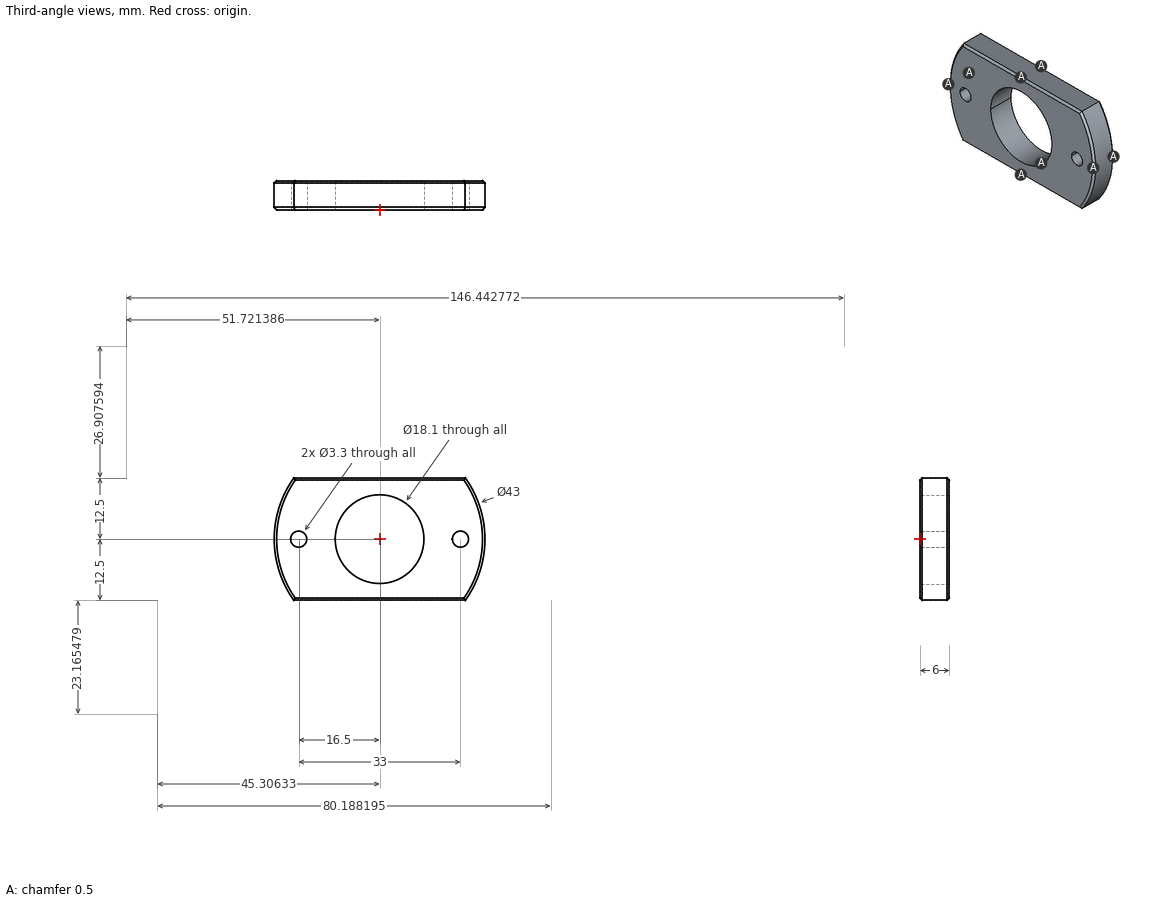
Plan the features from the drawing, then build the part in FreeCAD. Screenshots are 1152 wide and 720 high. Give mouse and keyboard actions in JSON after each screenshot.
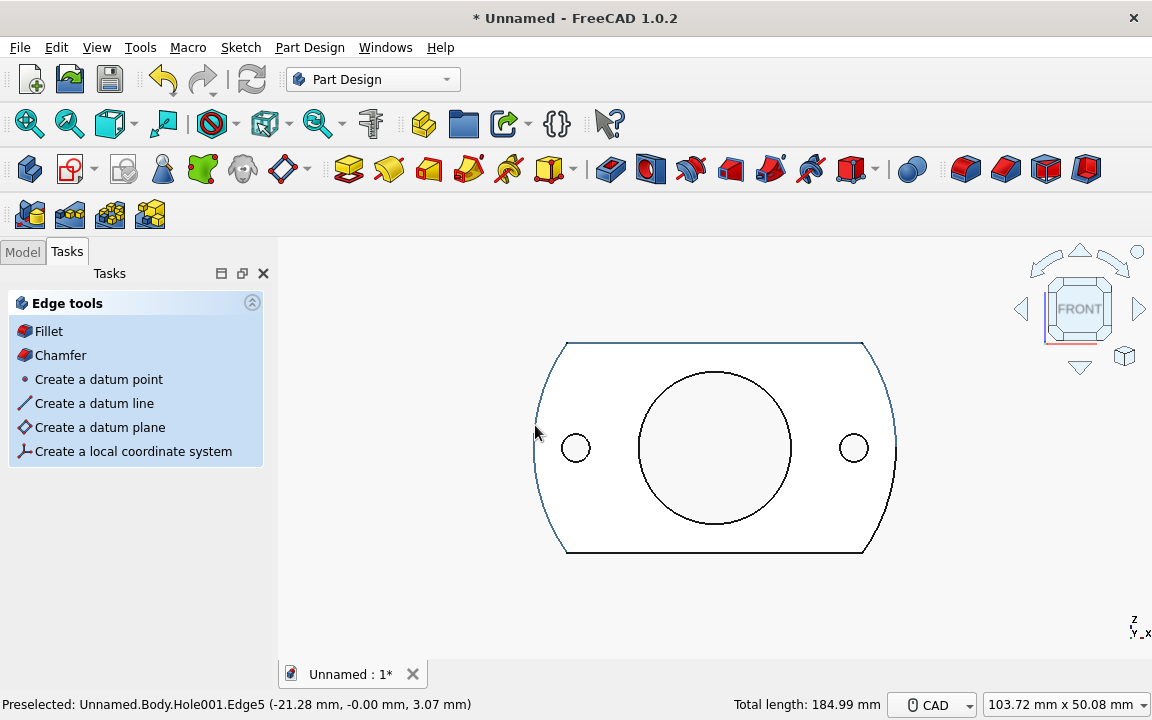
{"action": "key", "text": "3"}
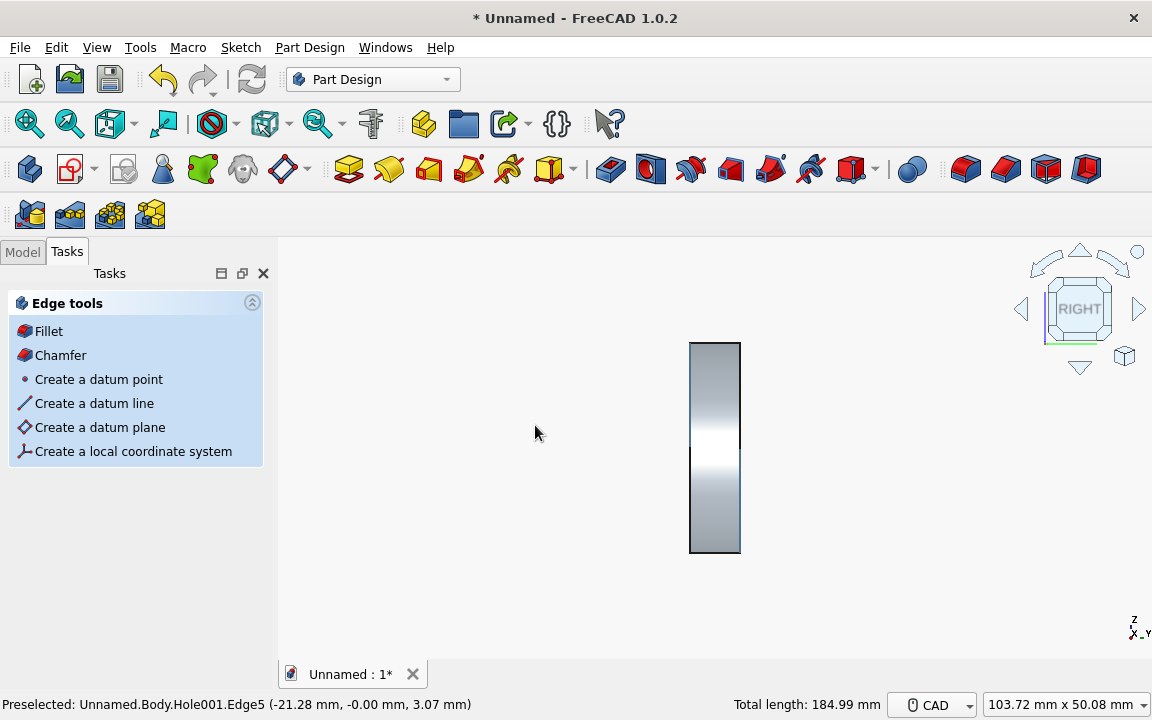
{"action": "key", "text": "5"}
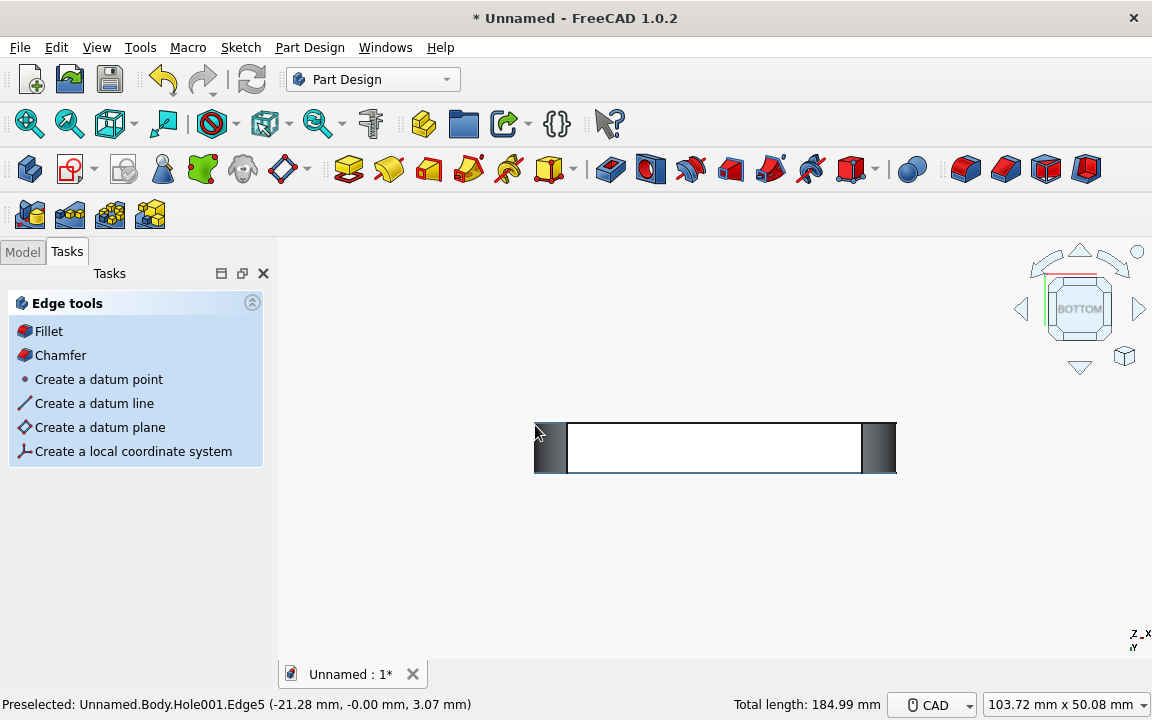
{"action": "left_click", "coordinate": [30, 124]}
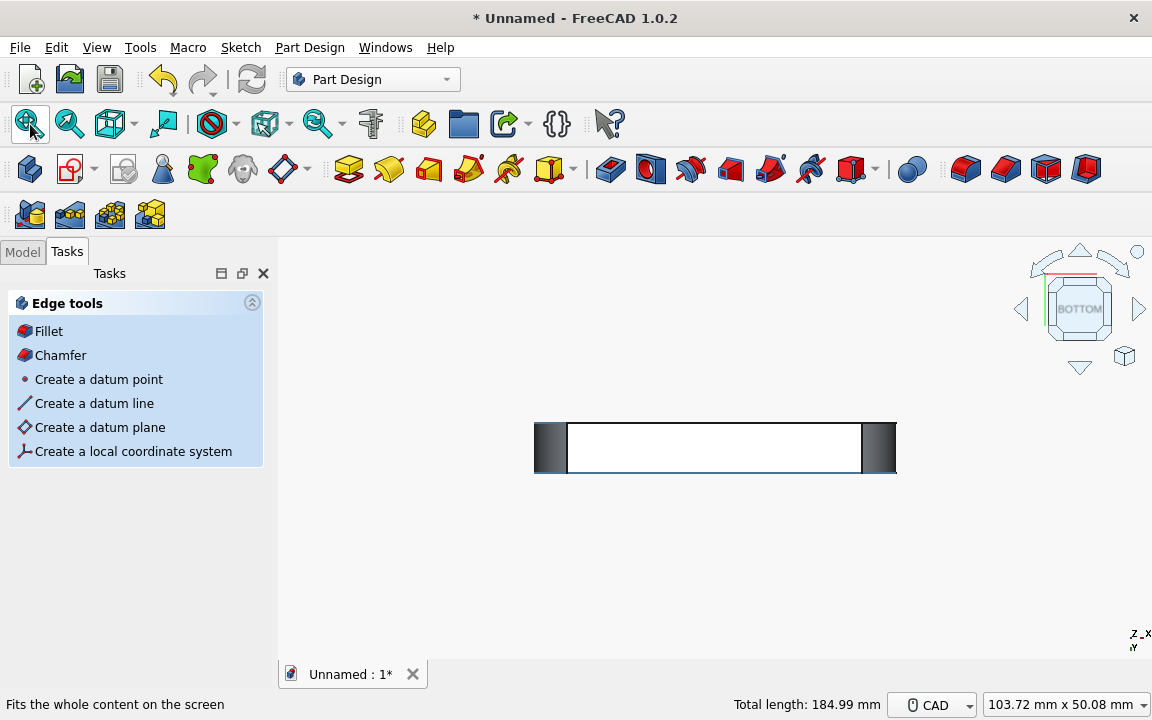
{"action": "left_click", "coordinate": [715, 422], "text": "ctrl"}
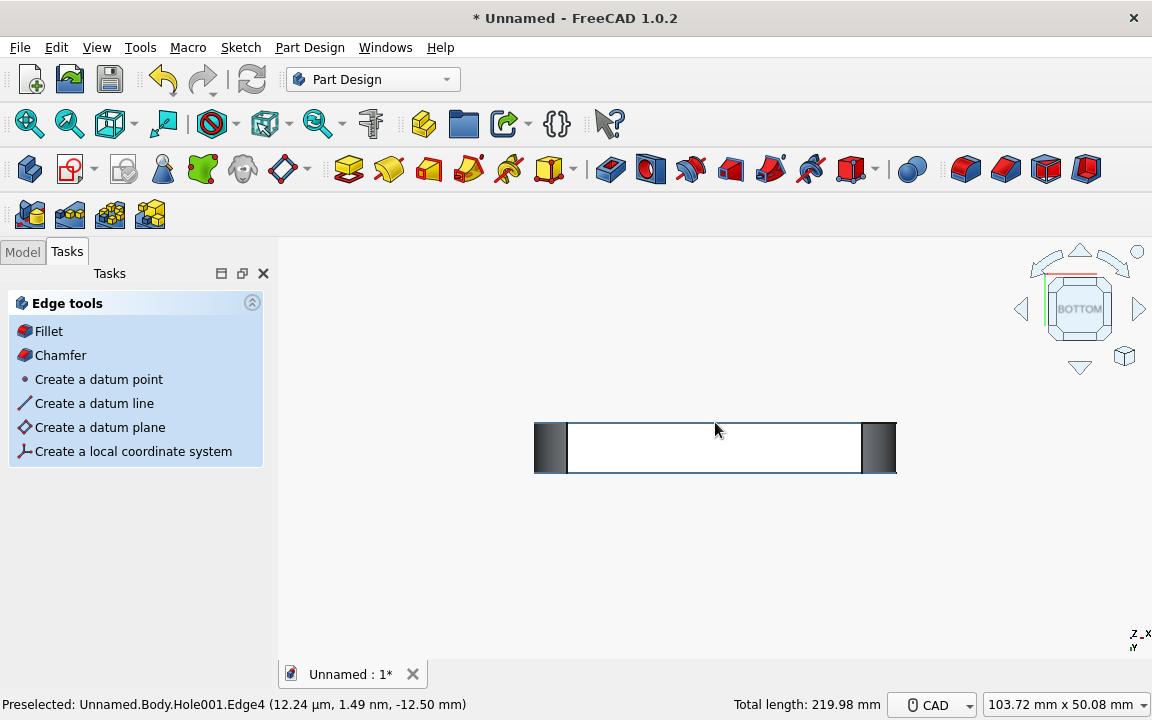
{"action": "left_click", "coordinate": [1006, 170]}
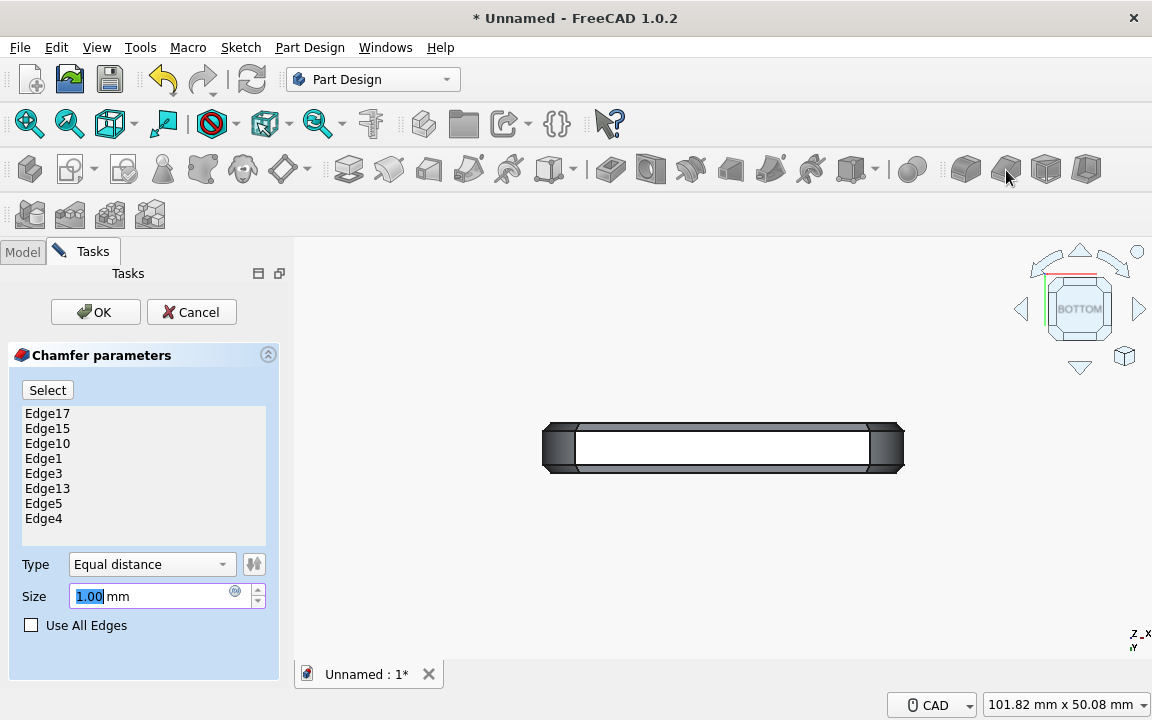
{"action": "type", "text": "0.5"}
{"action": "key", "text": "Tab"}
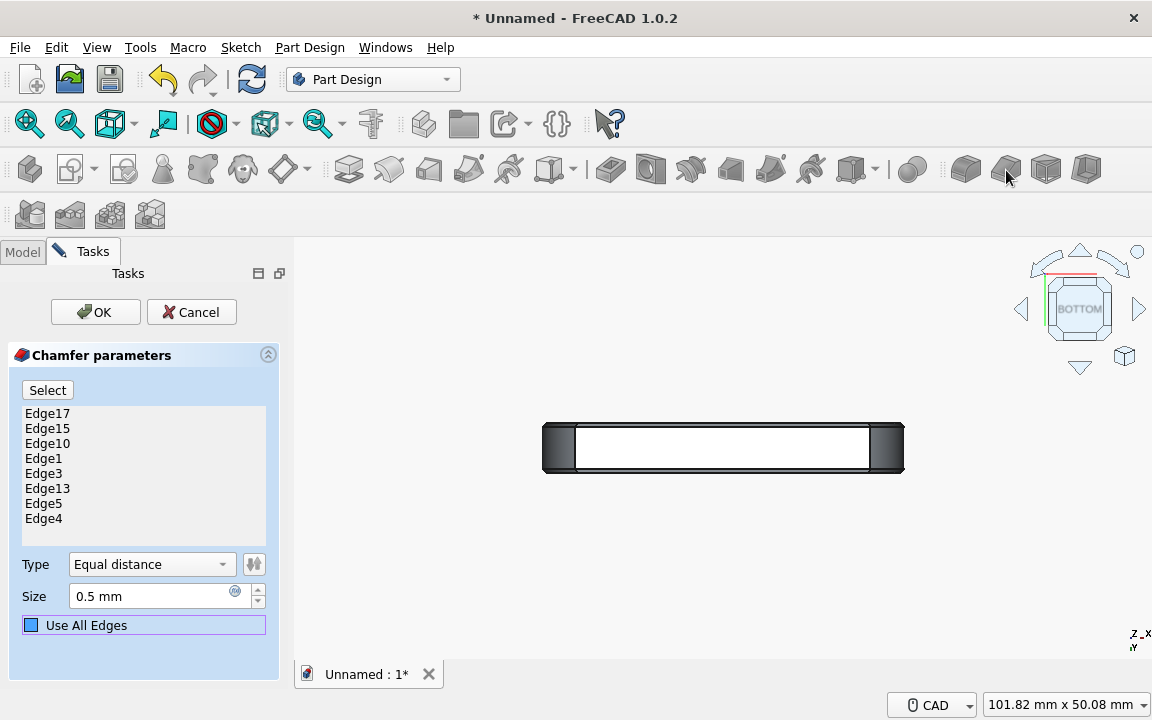
{"action": "left_click", "coordinate": [96, 312]}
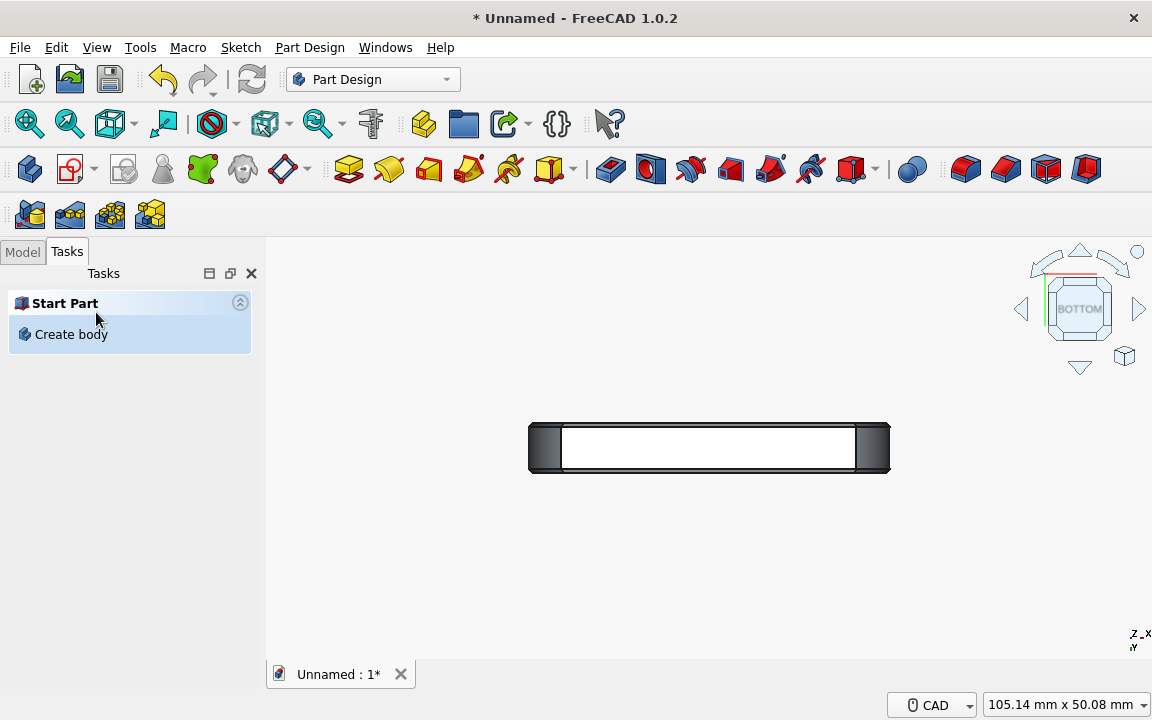
{"action": "key", "text": "0"}